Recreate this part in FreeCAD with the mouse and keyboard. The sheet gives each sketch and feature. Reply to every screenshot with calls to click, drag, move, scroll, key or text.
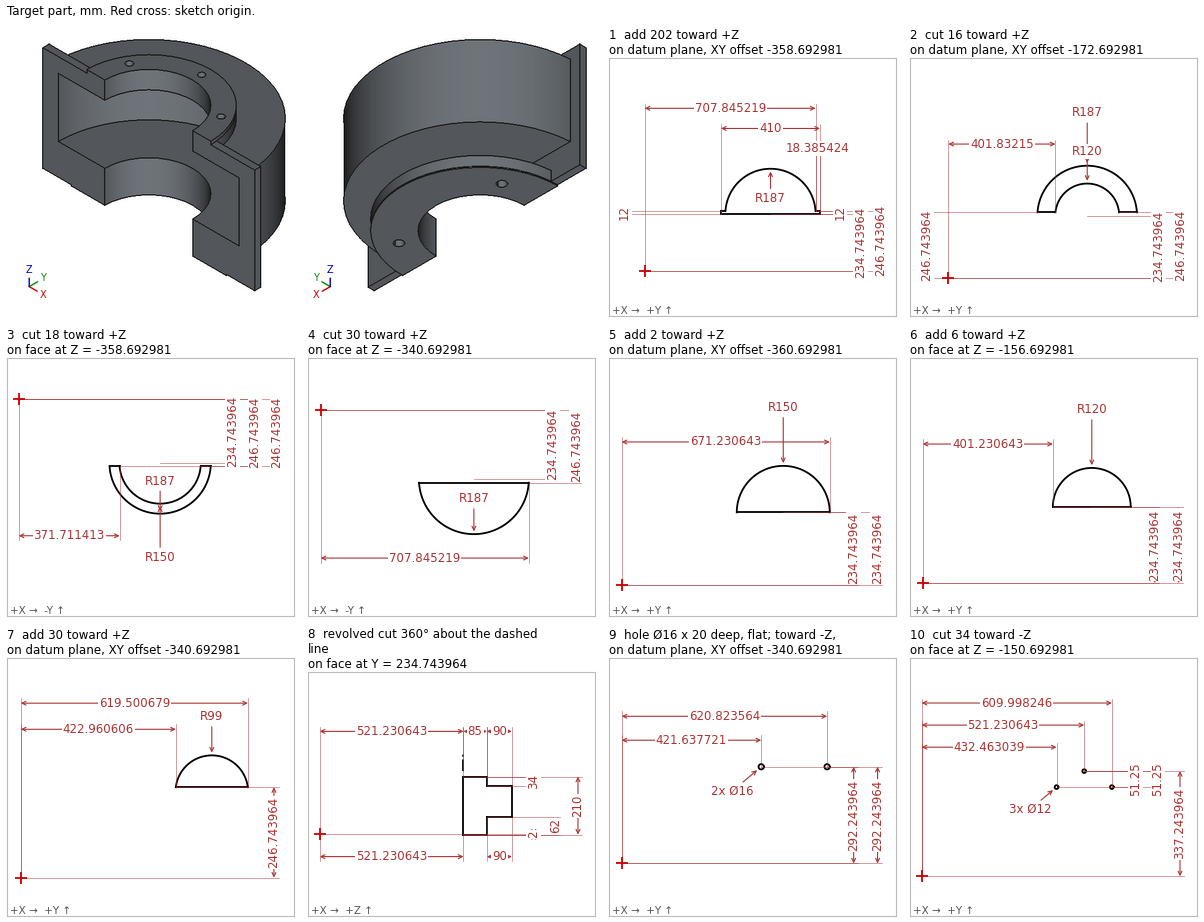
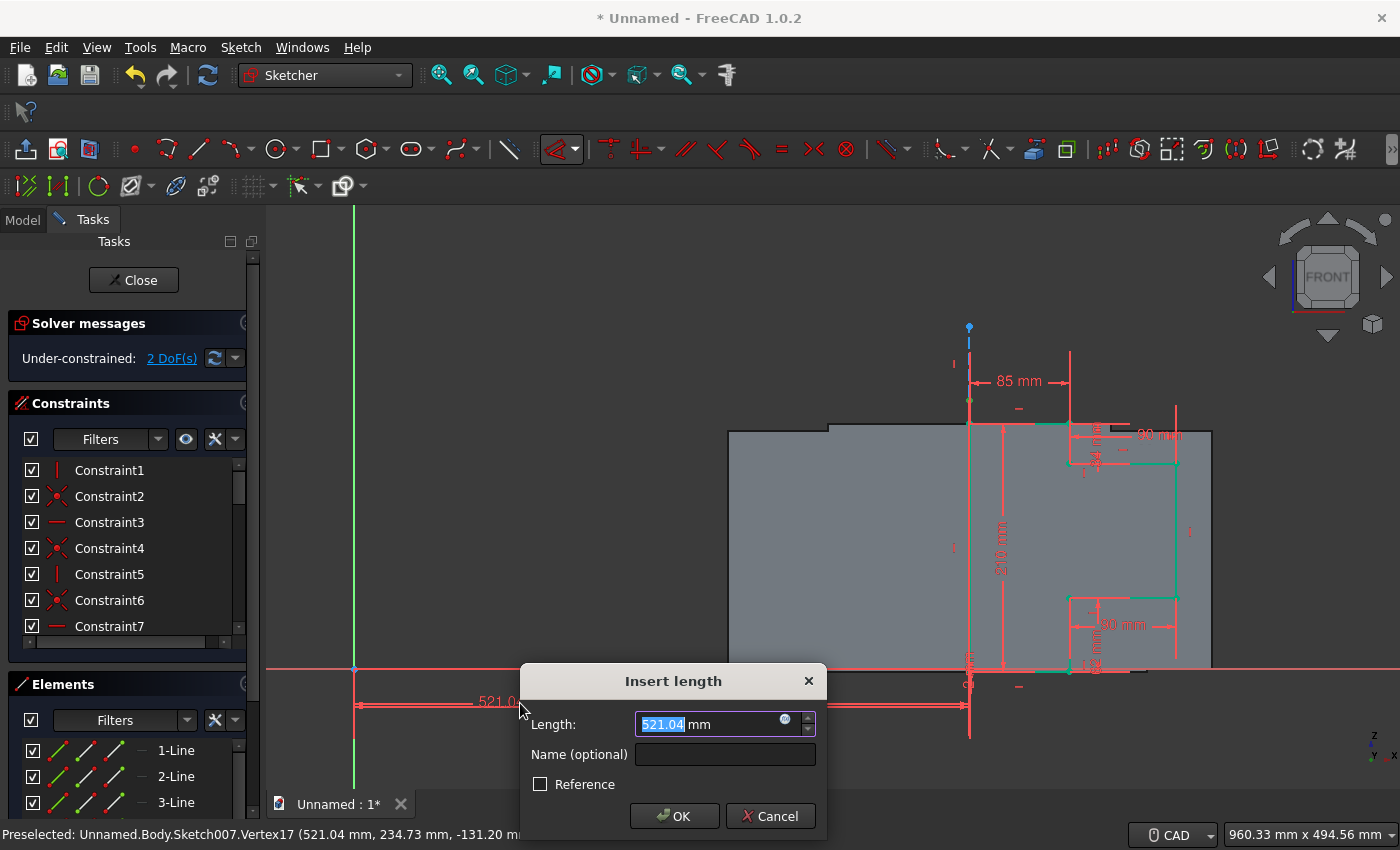
text(521.230643)
key(Return)
key(Escape)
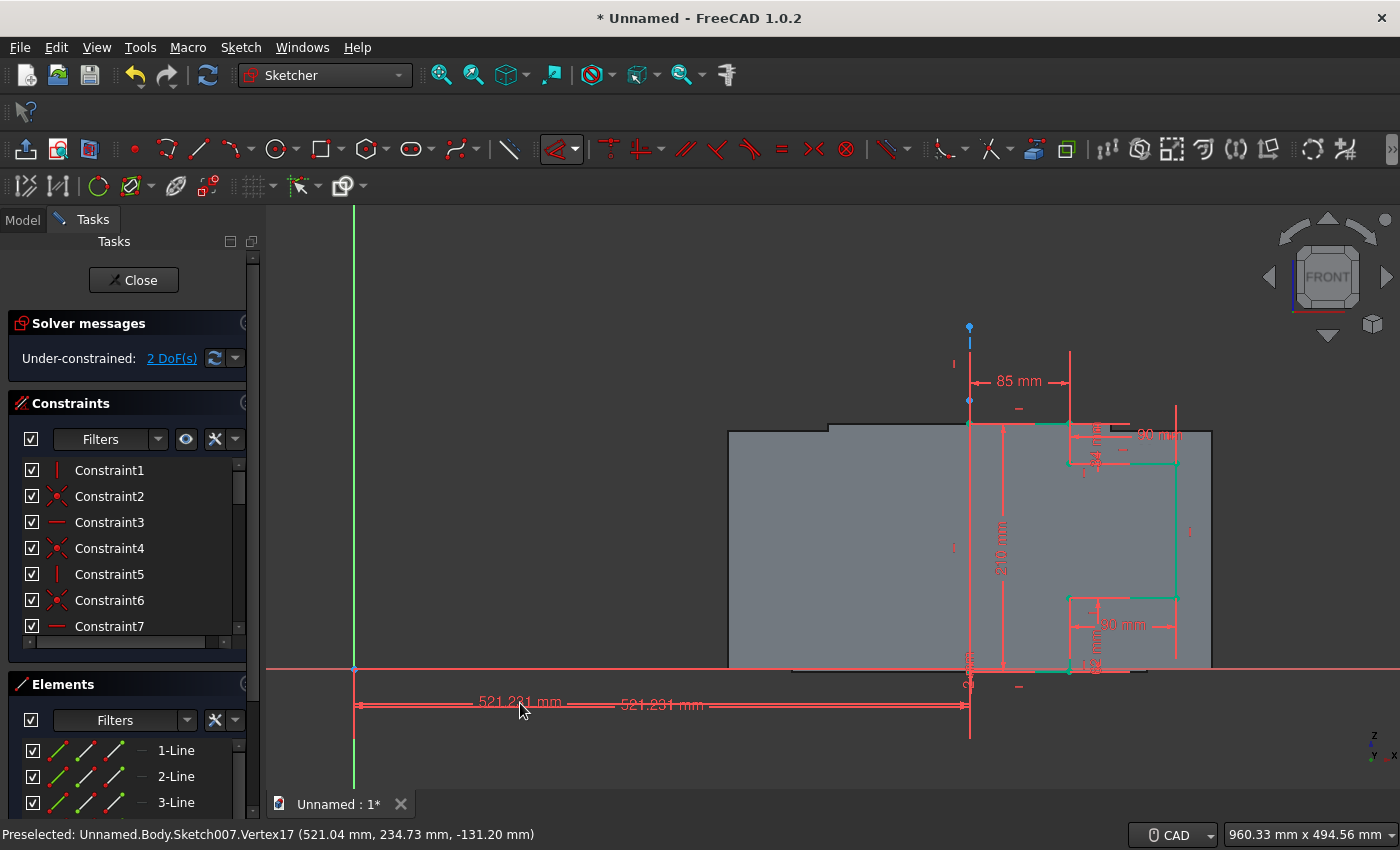
click(134, 280)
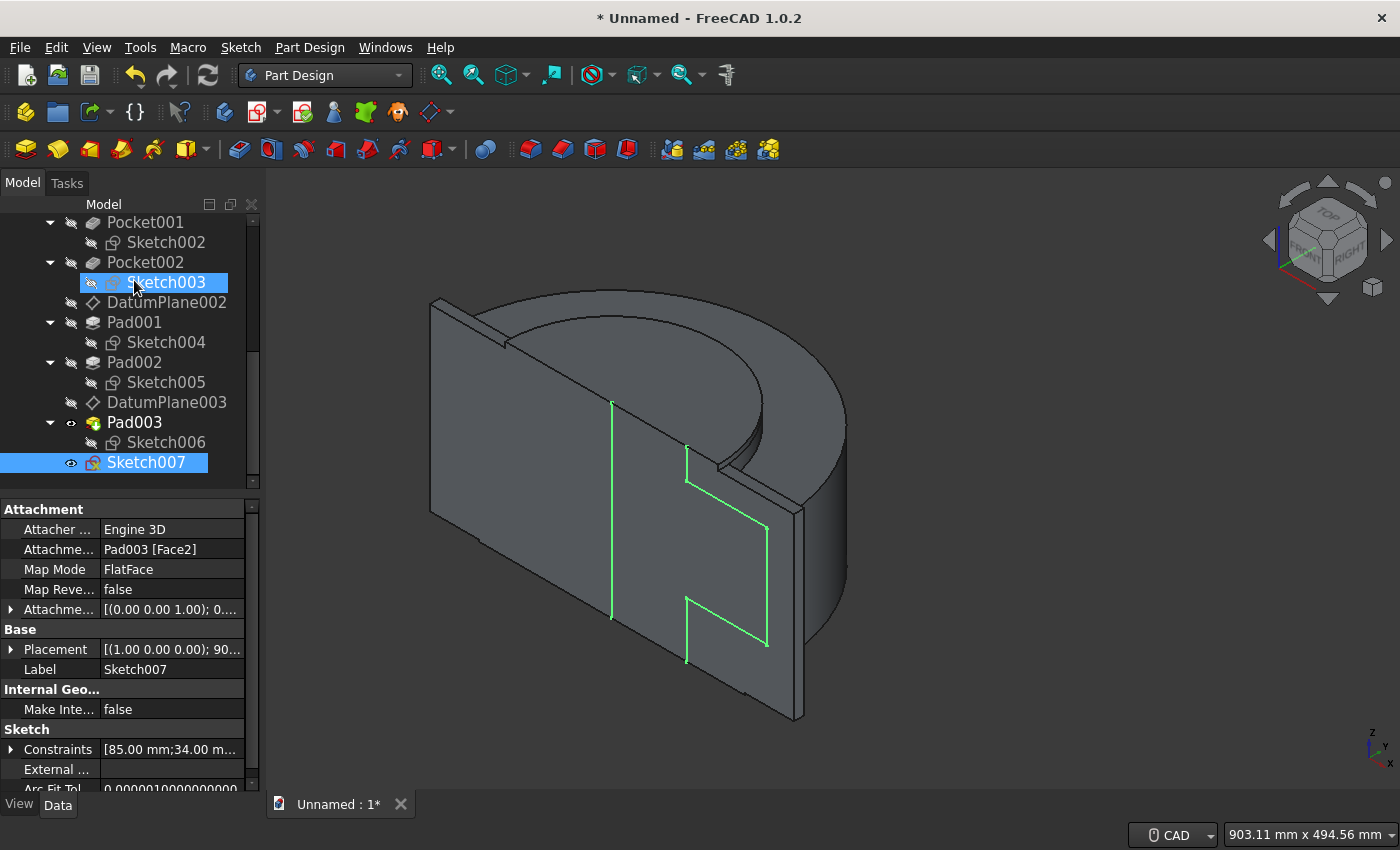
click(304, 150)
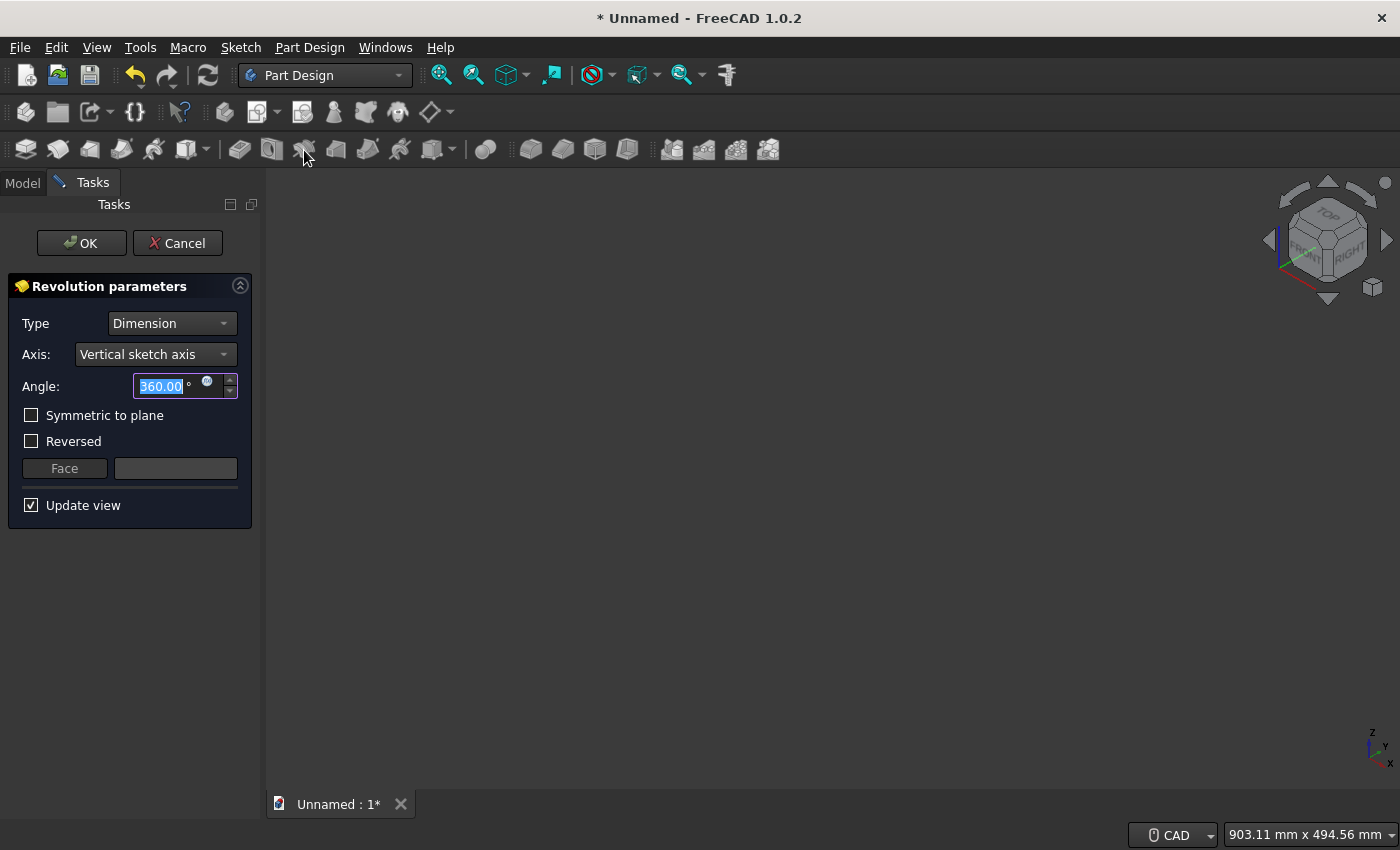
click(156, 354)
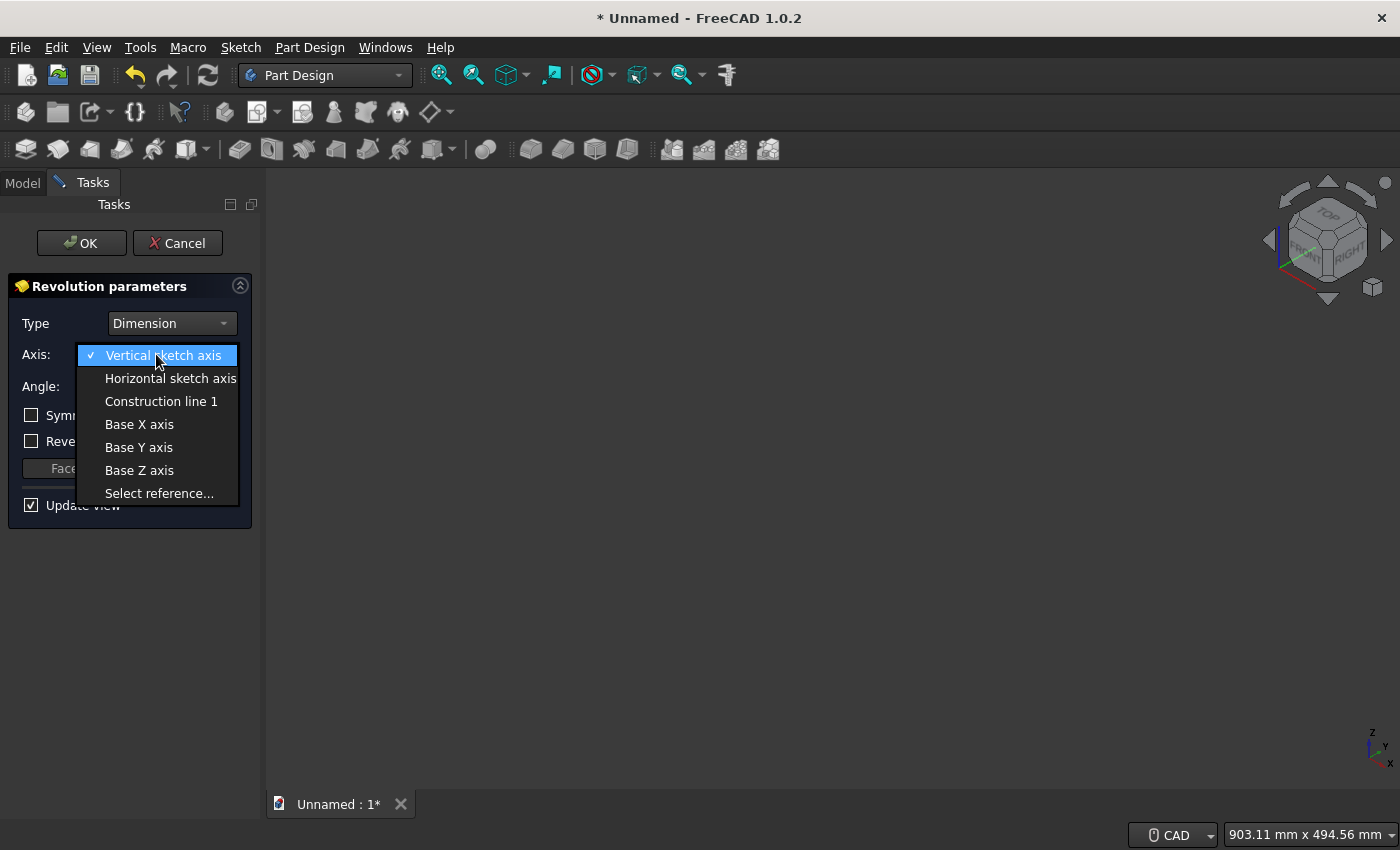
click(156, 402)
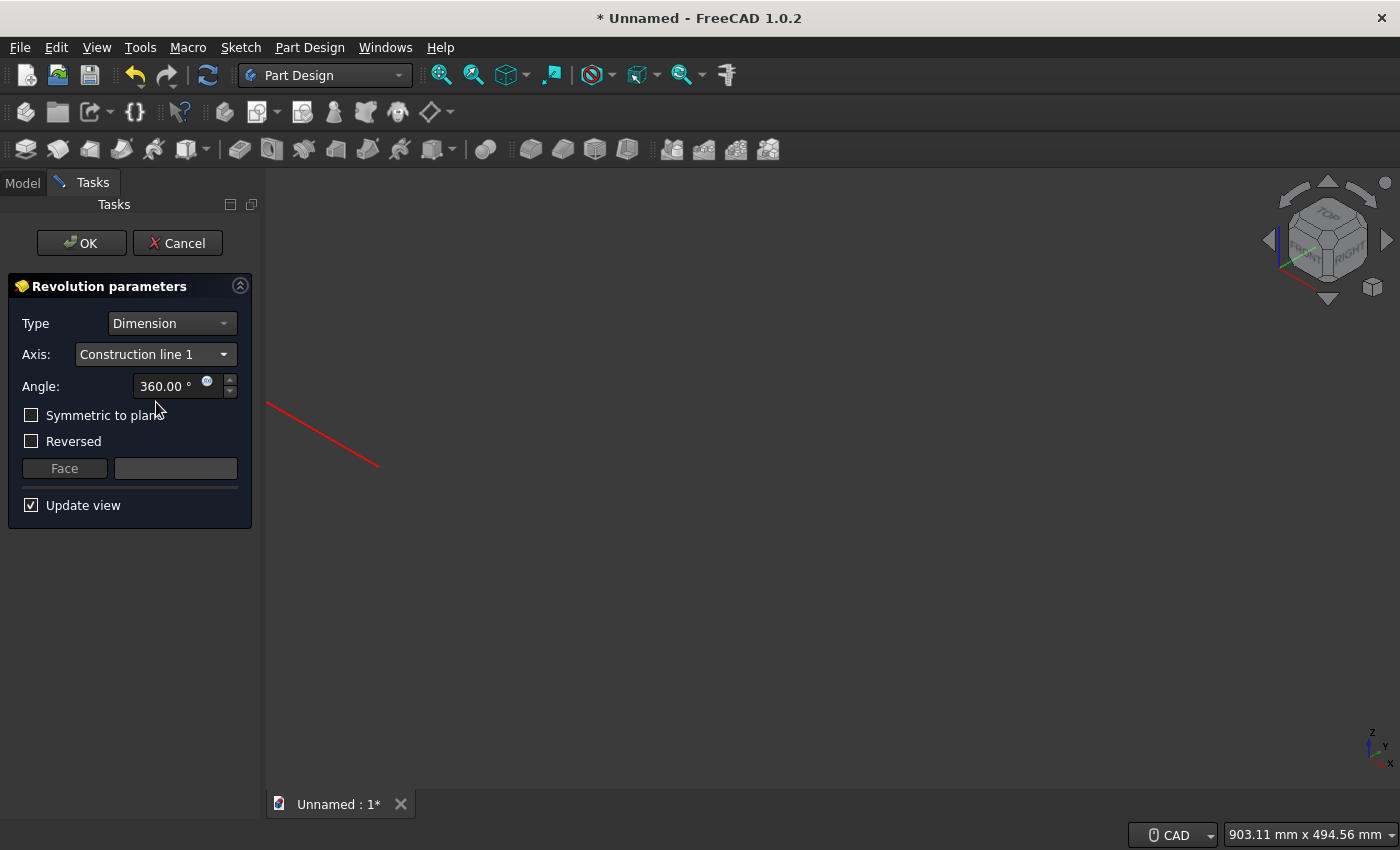
click(82, 243)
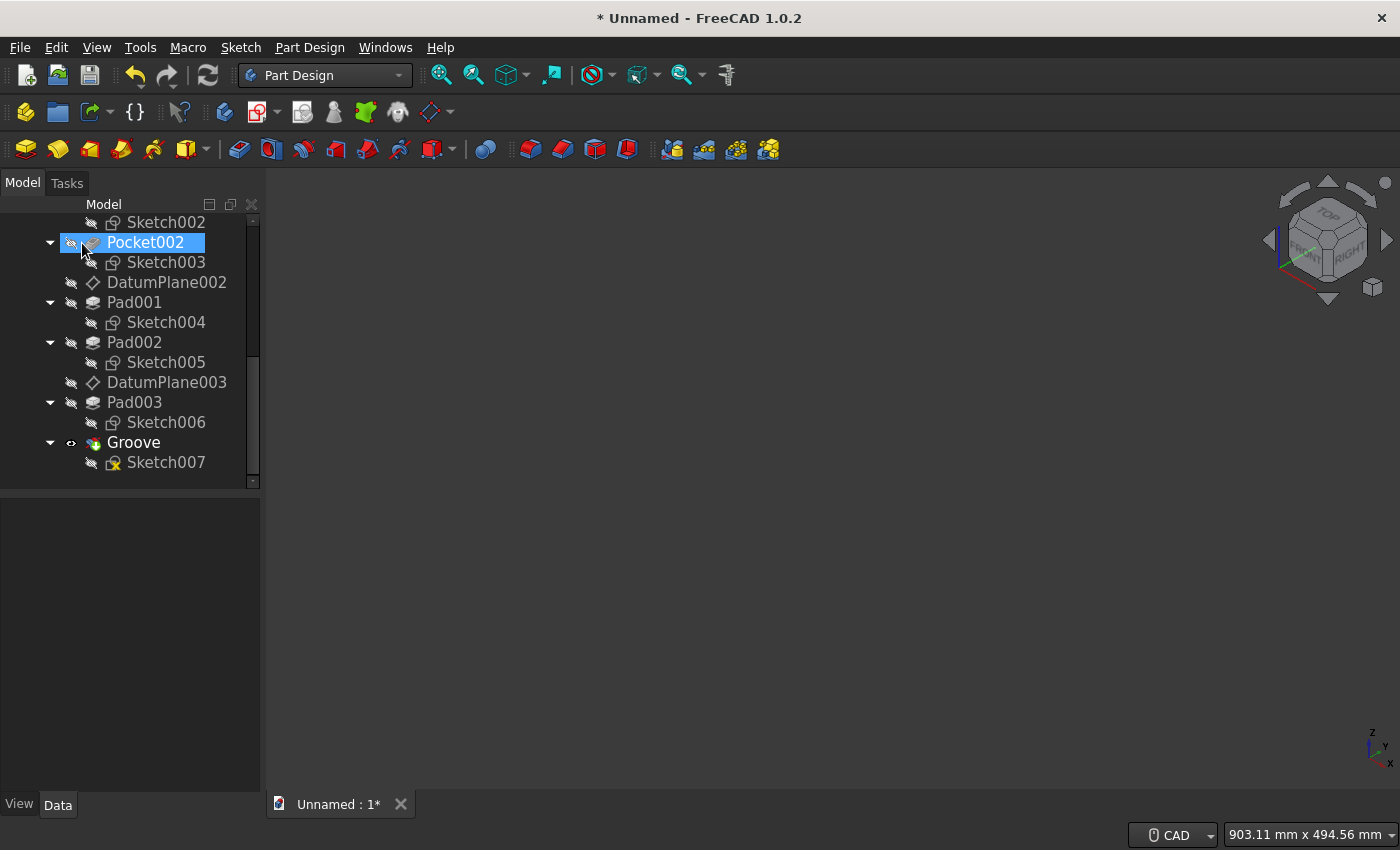
key(v)
key(f)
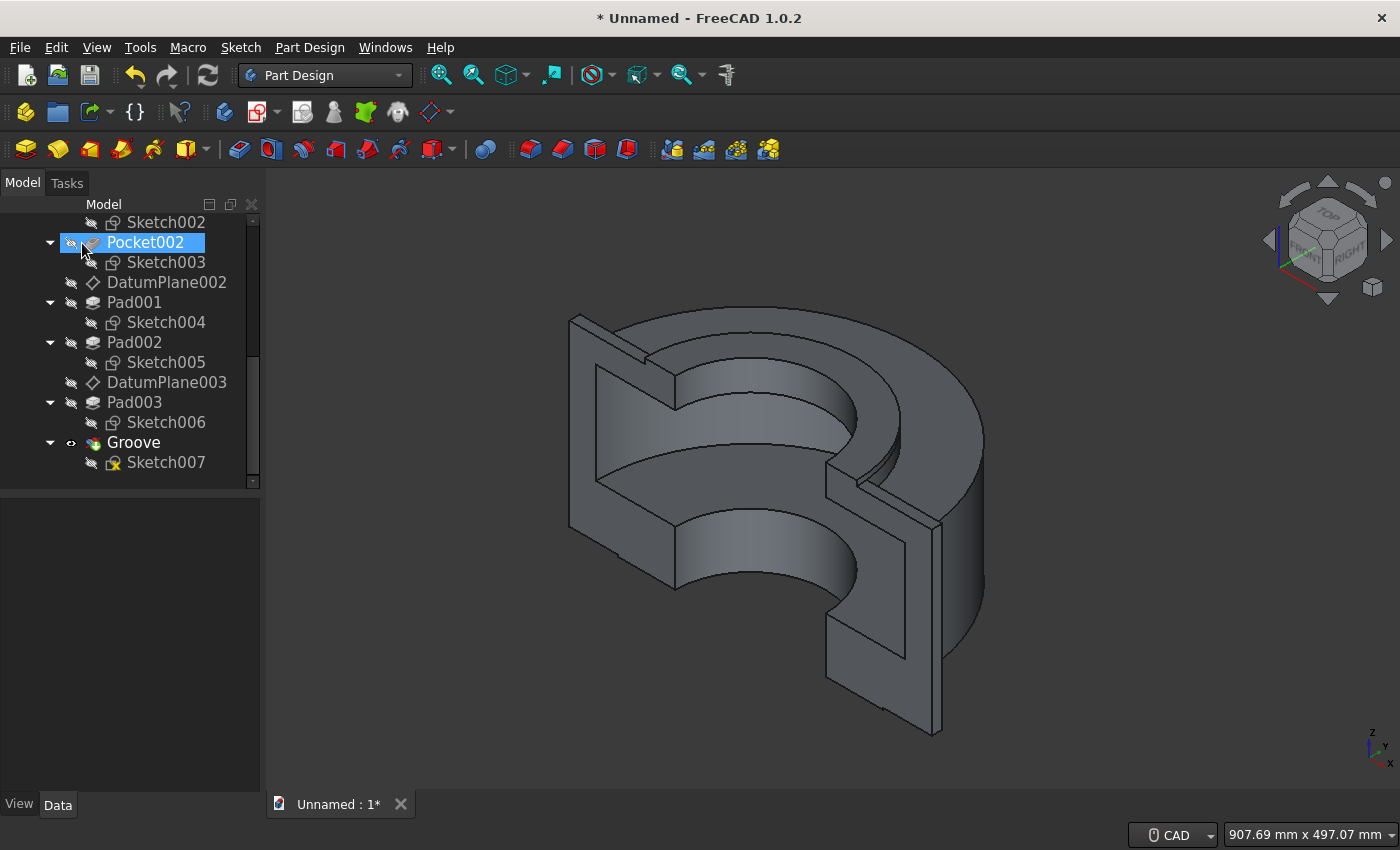
scroll(160, 338, down, 3)